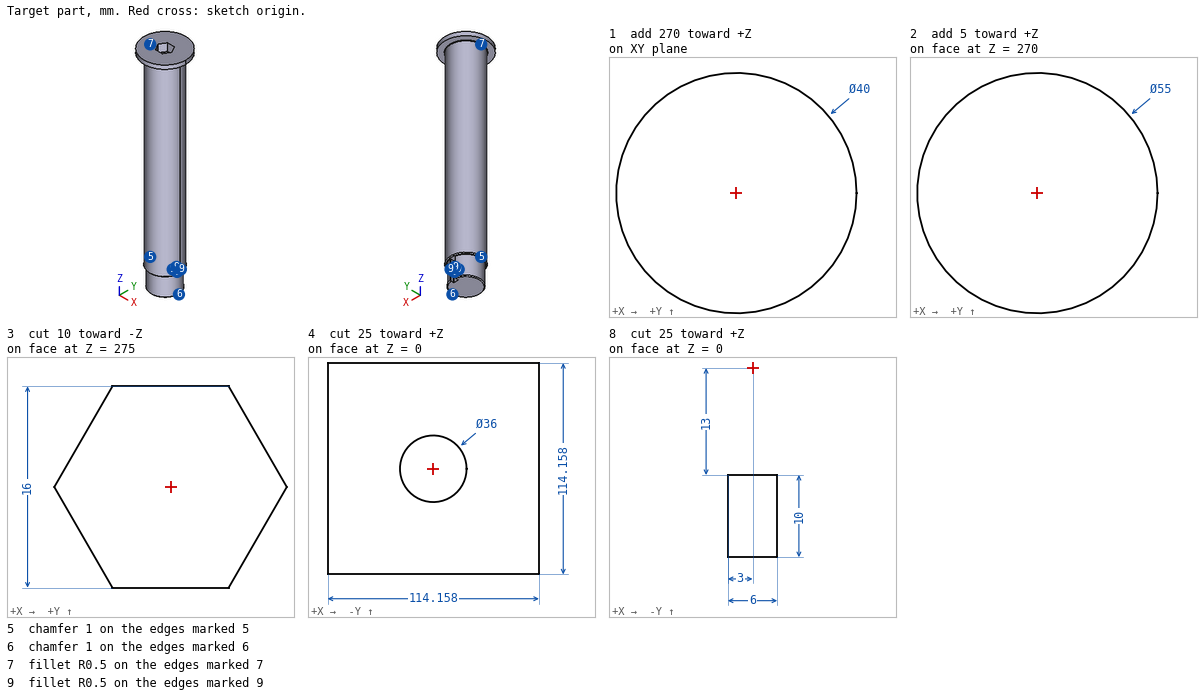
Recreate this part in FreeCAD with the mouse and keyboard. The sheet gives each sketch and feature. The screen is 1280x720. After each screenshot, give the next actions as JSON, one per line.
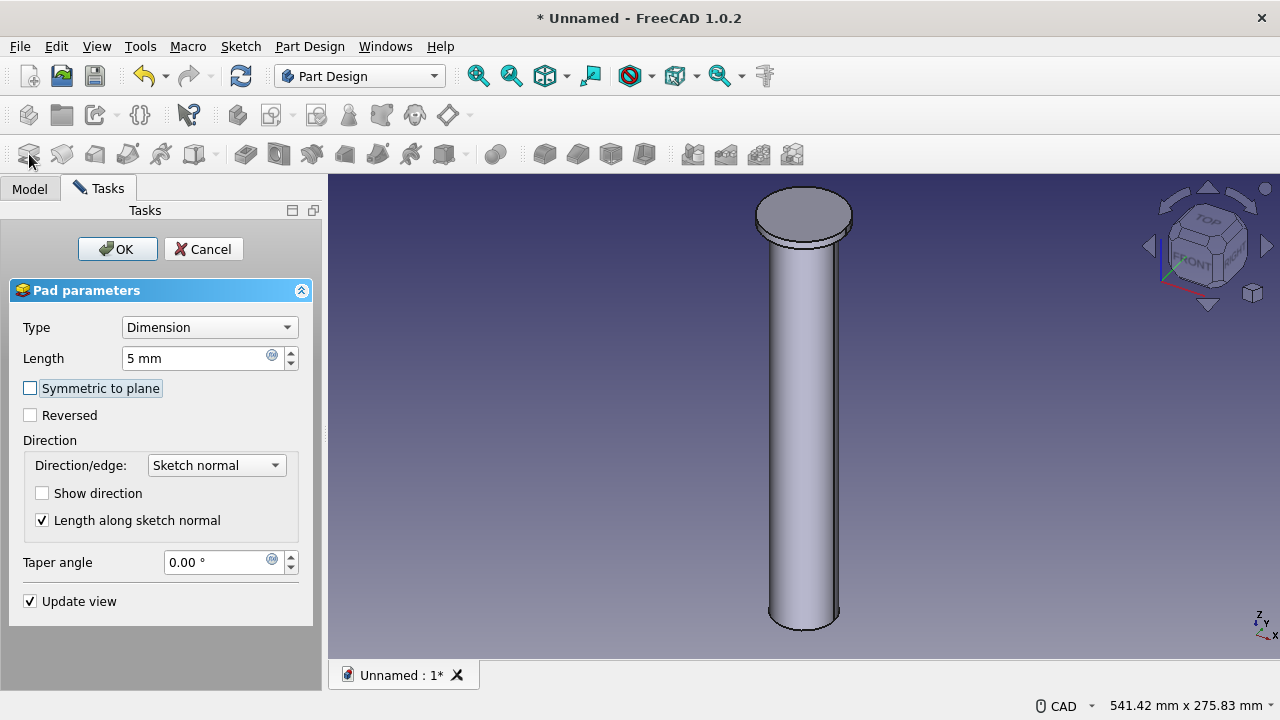
{"action": "left_click", "coordinate": [118, 249]}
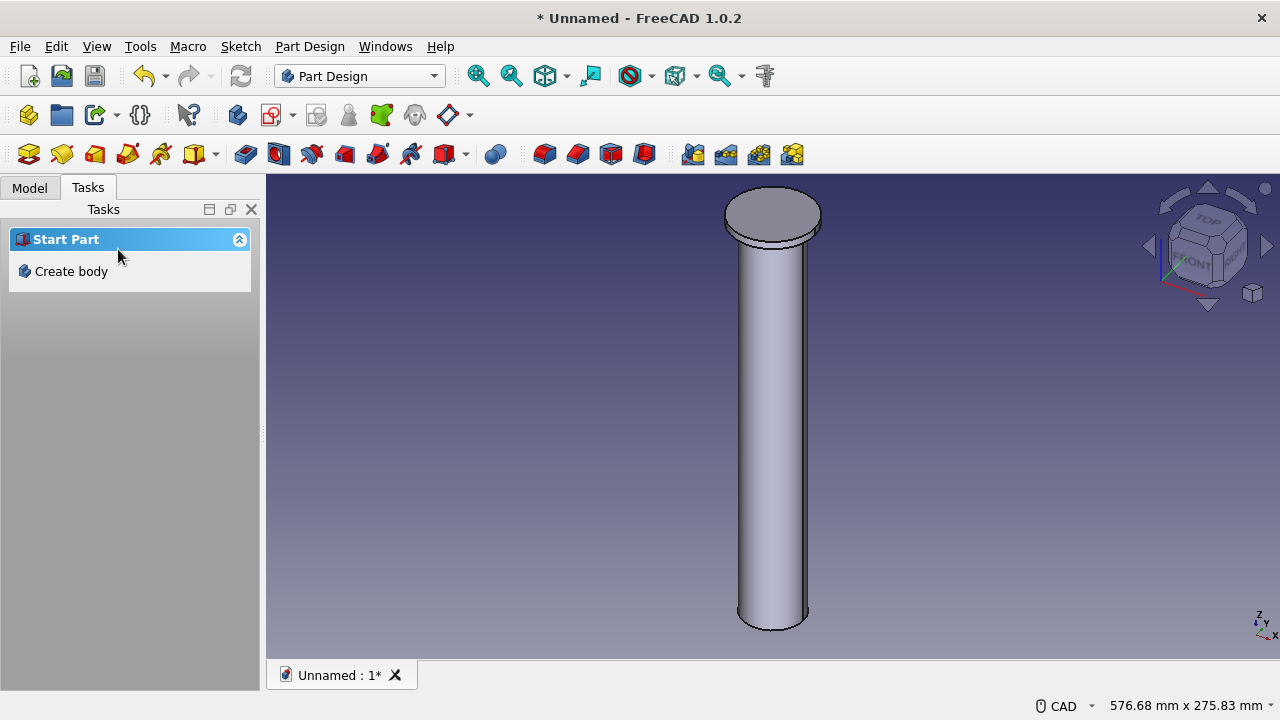
{"action": "left_click", "coordinate": [773, 213]}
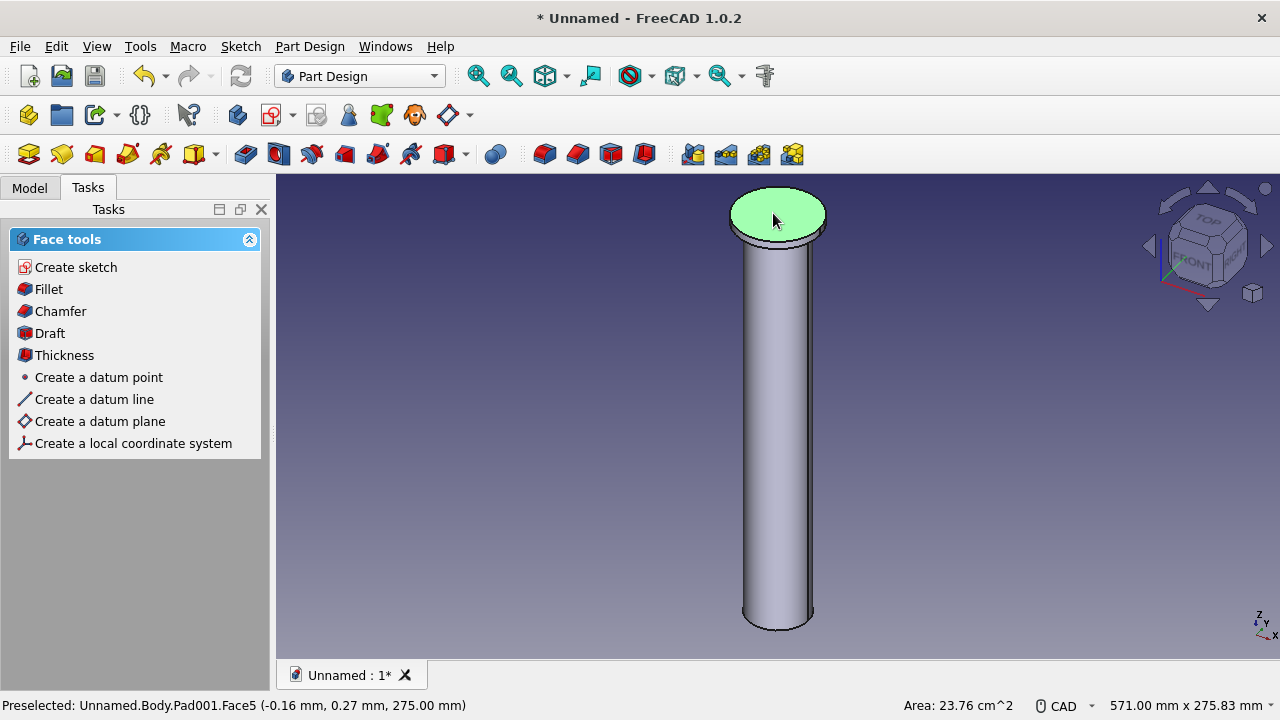
{"action": "left_click", "coordinate": [270, 116]}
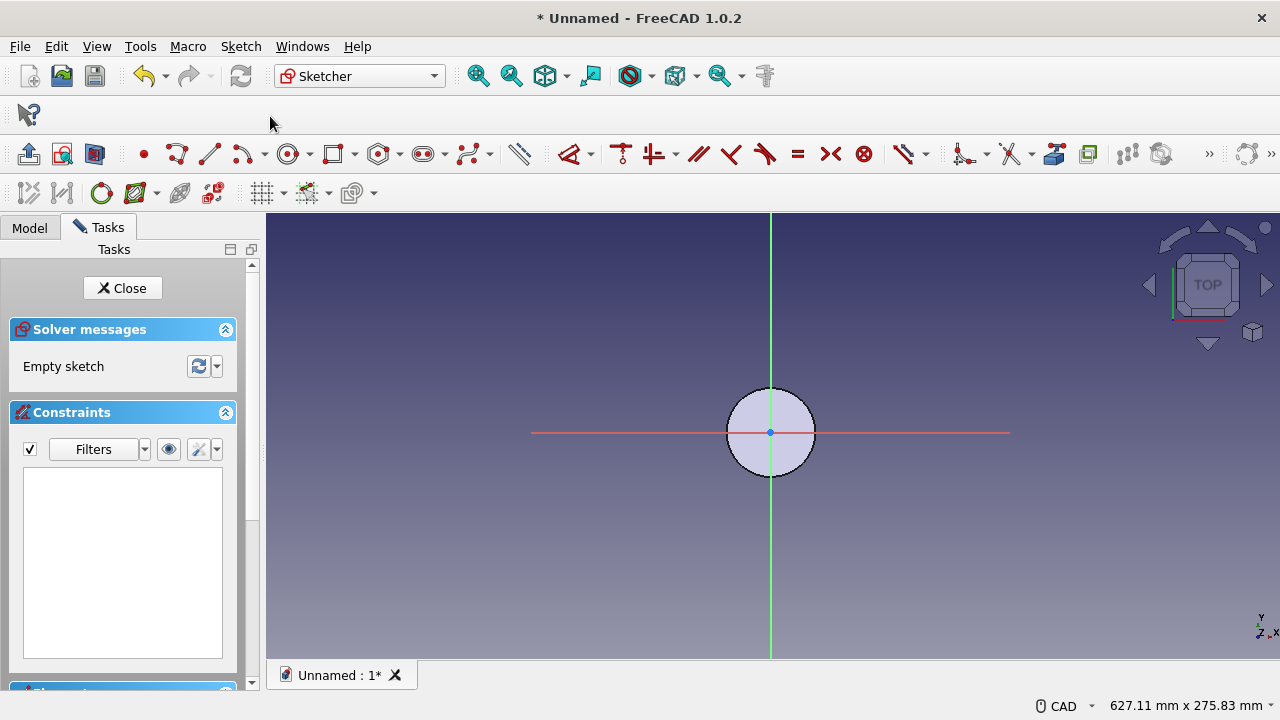
{"action": "scroll", "coordinate": [778, 432], "scroll_direction": "up", "scroll_amount": 12}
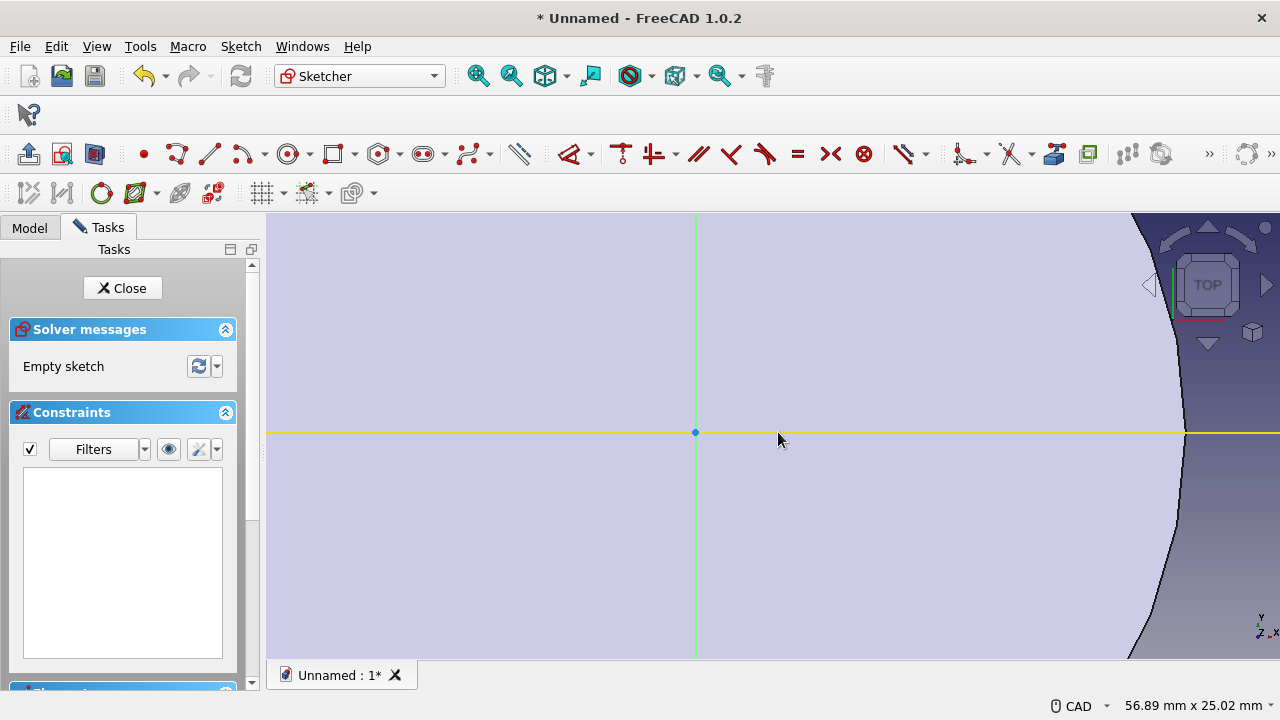
{"action": "left_click", "coordinate": [378, 154]}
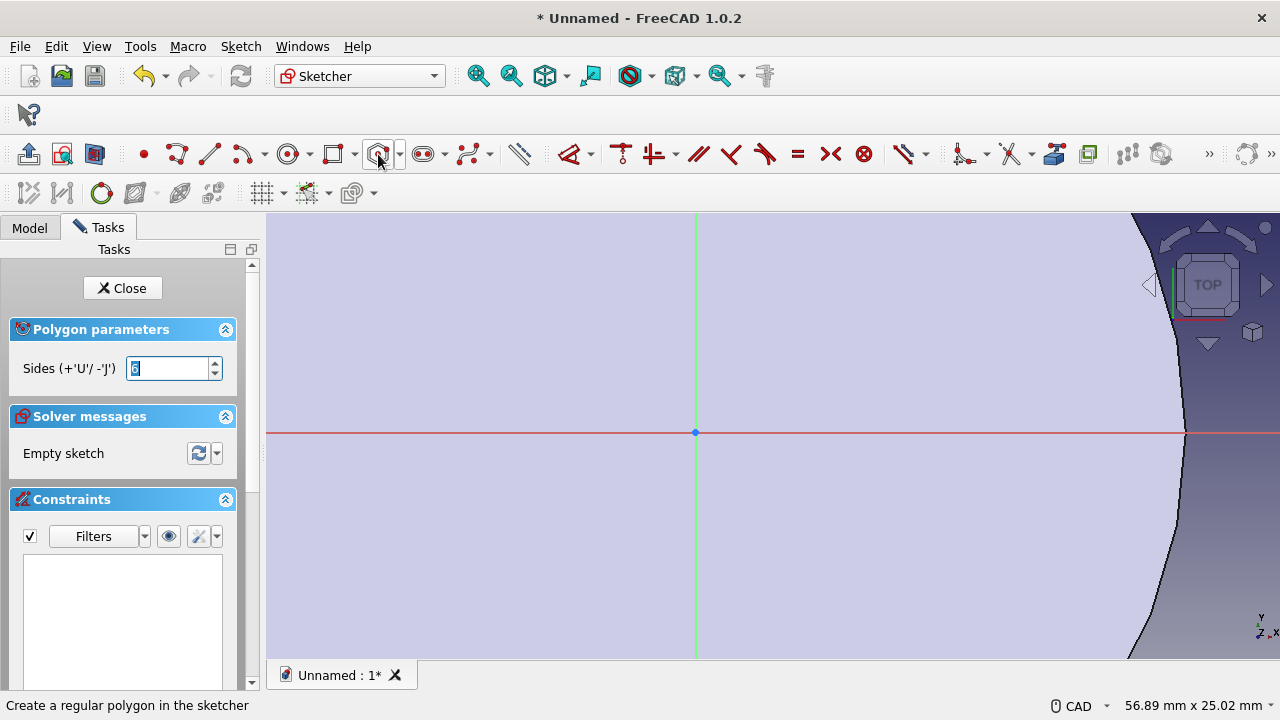
{"action": "left_click", "coordinate": [696, 433]}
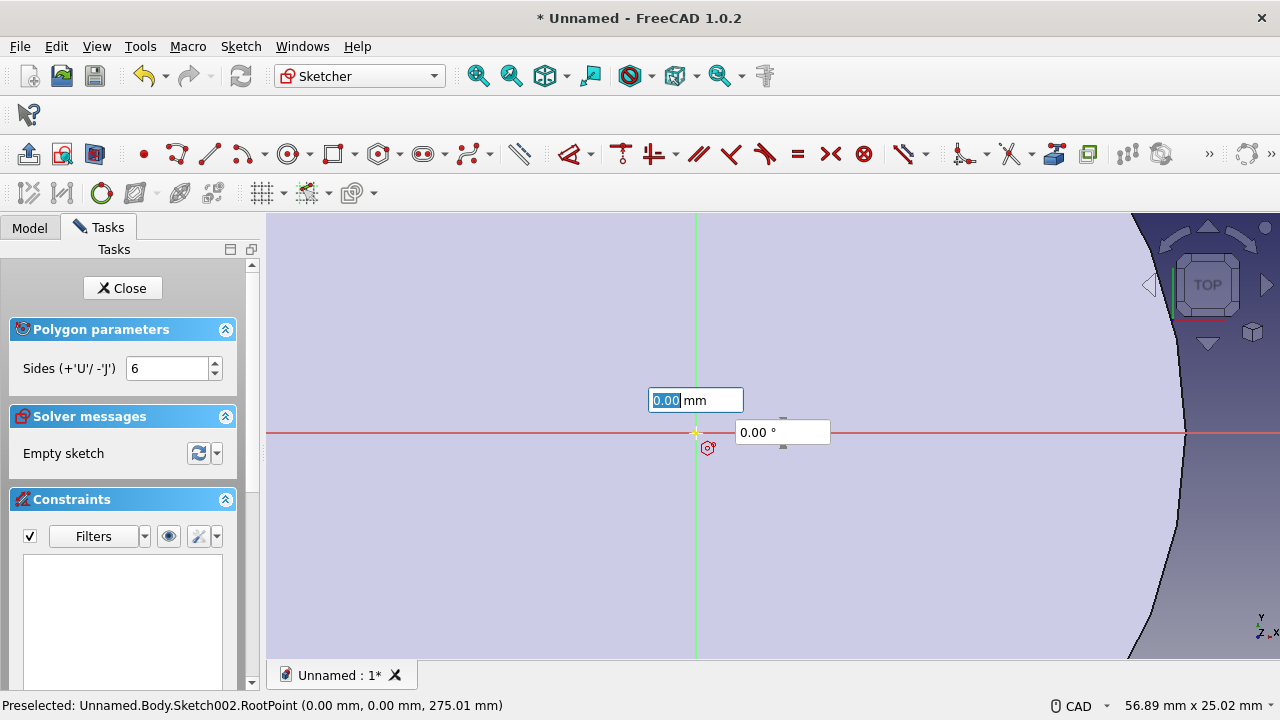
{"action": "left_click", "coordinate": [860, 433]}
{"action": "right_click", "coordinate": [860, 433]}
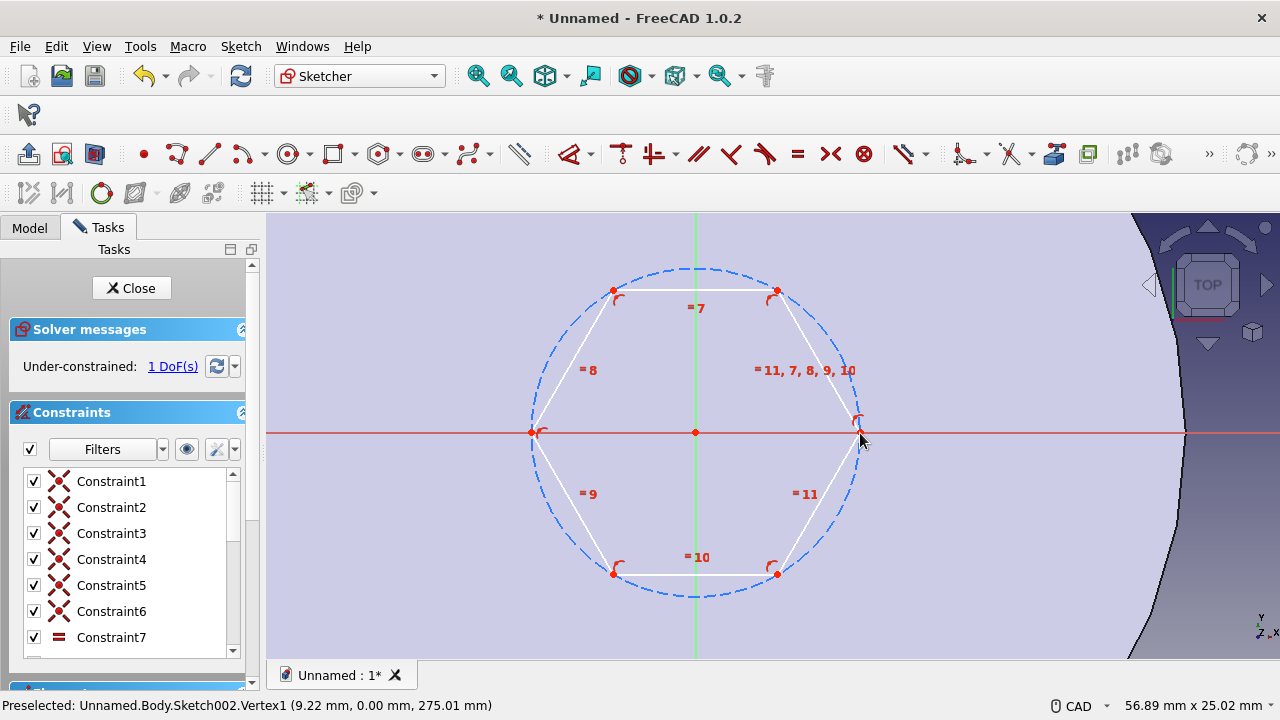
{"action": "left_click", "coordinate": [568, 154]}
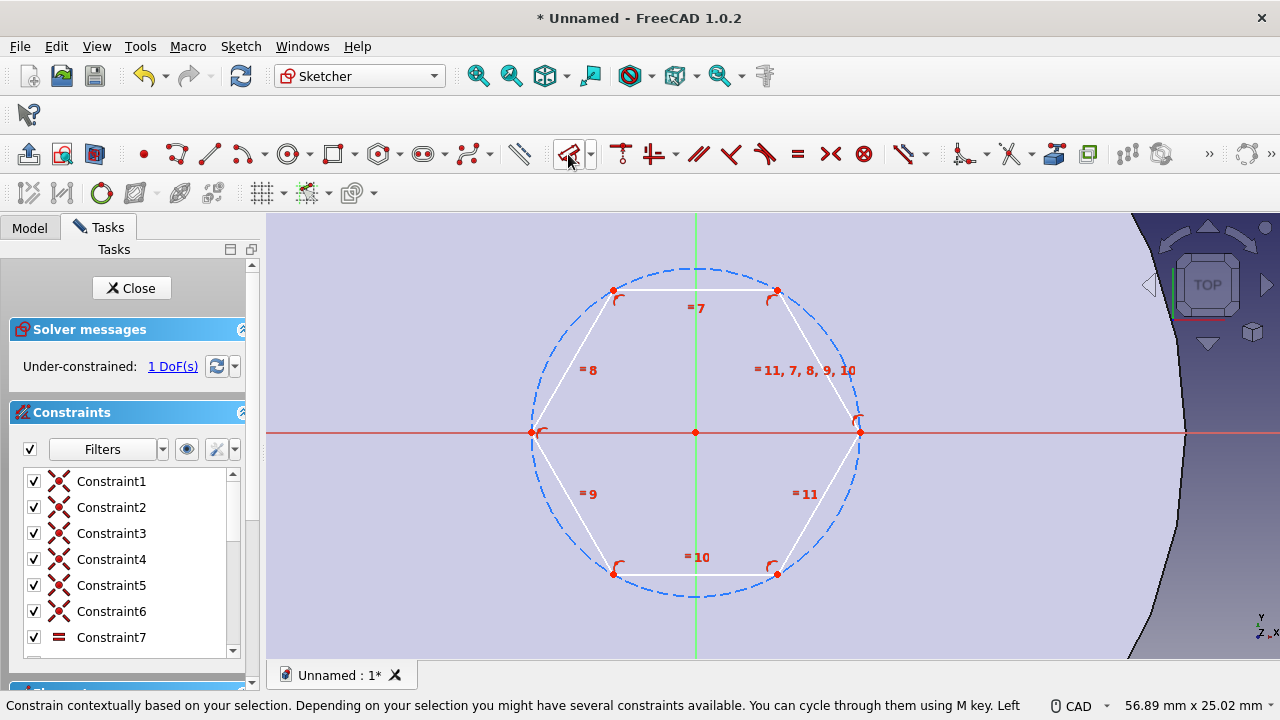
{"action": "left_click", "coordinate": [614, 575]}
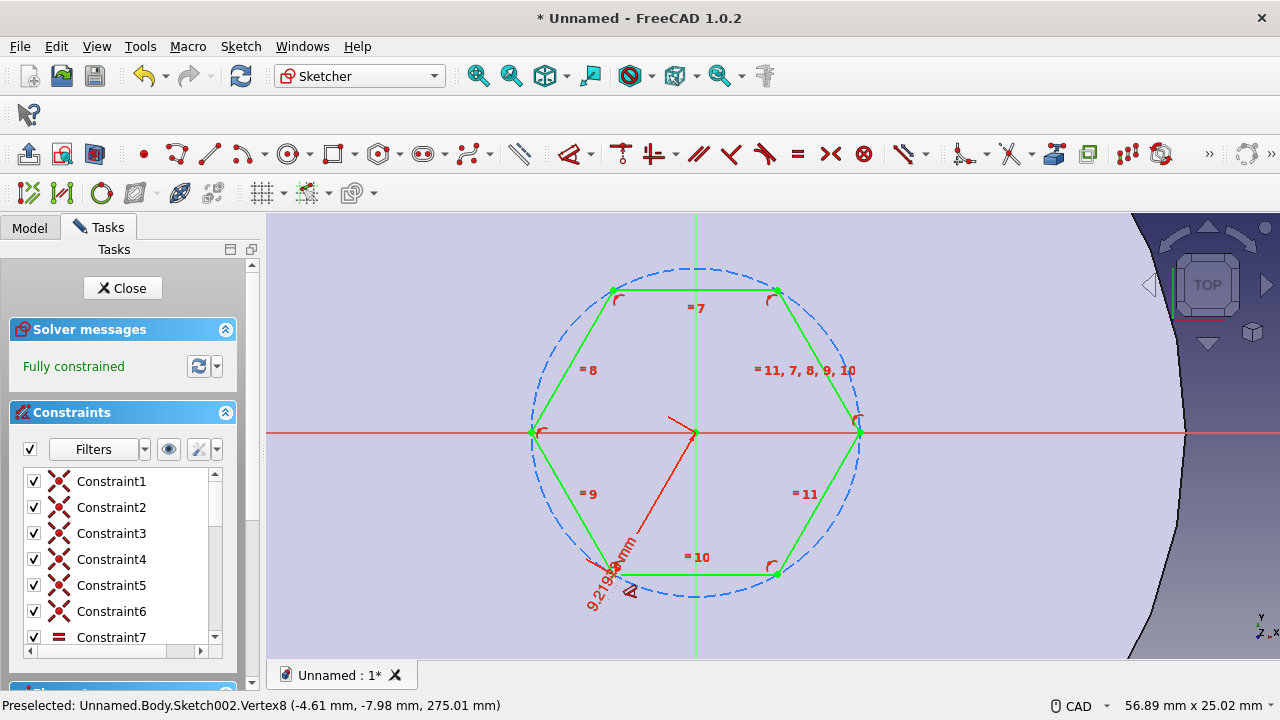
{"action": "left_click", "coordinate": [778, 290]}
{"action": "left_click", "coordinate": [860, 333]}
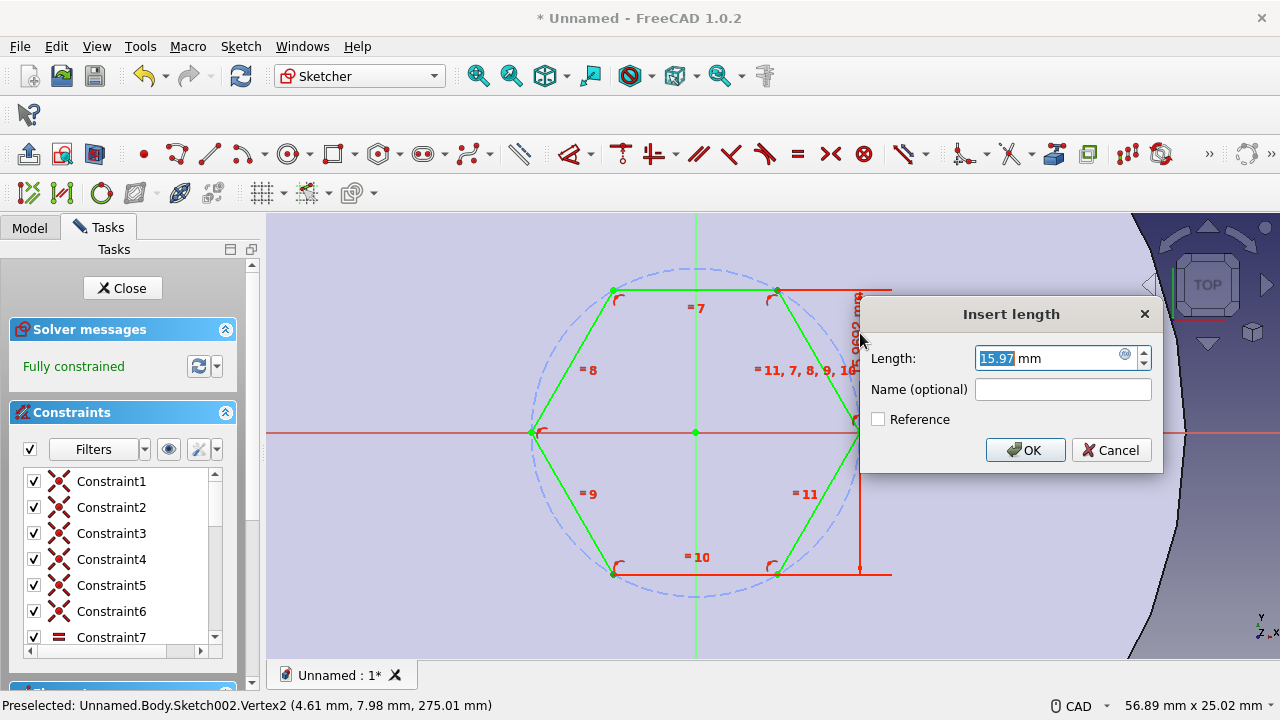
{"action": "type", "text": "16"}
{"action": "key", "text": "Return"}
{"action": "key", "text": "Escape"}